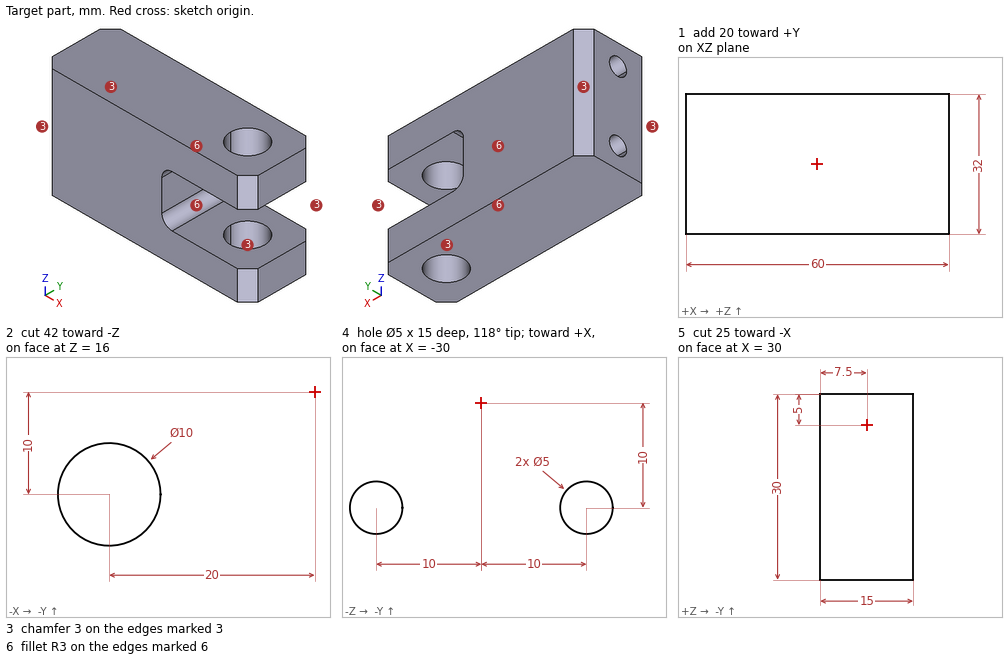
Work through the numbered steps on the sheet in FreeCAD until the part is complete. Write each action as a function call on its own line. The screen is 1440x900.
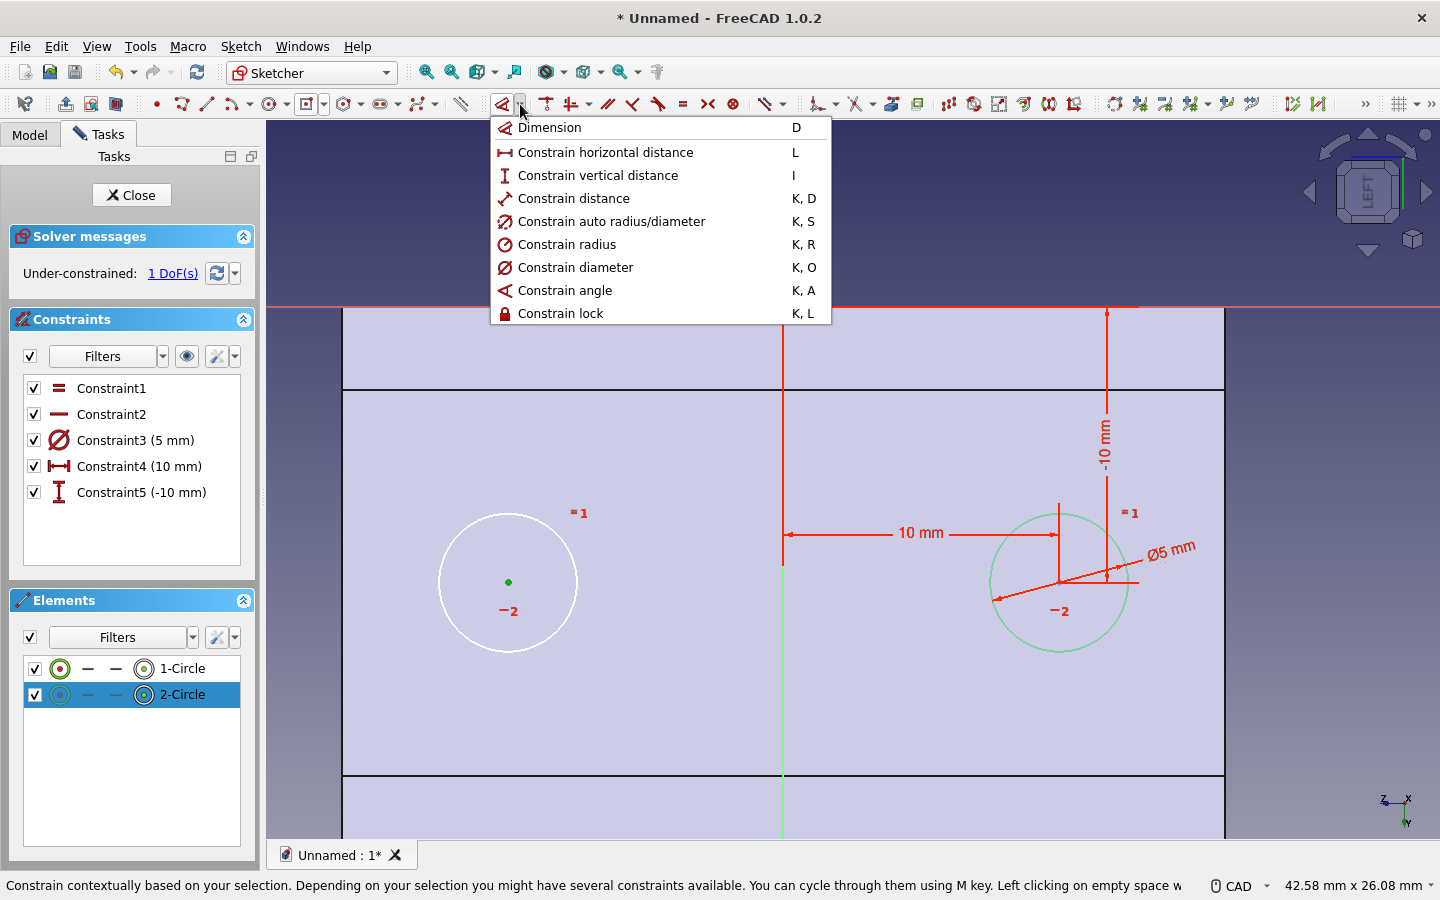
click(661, 152)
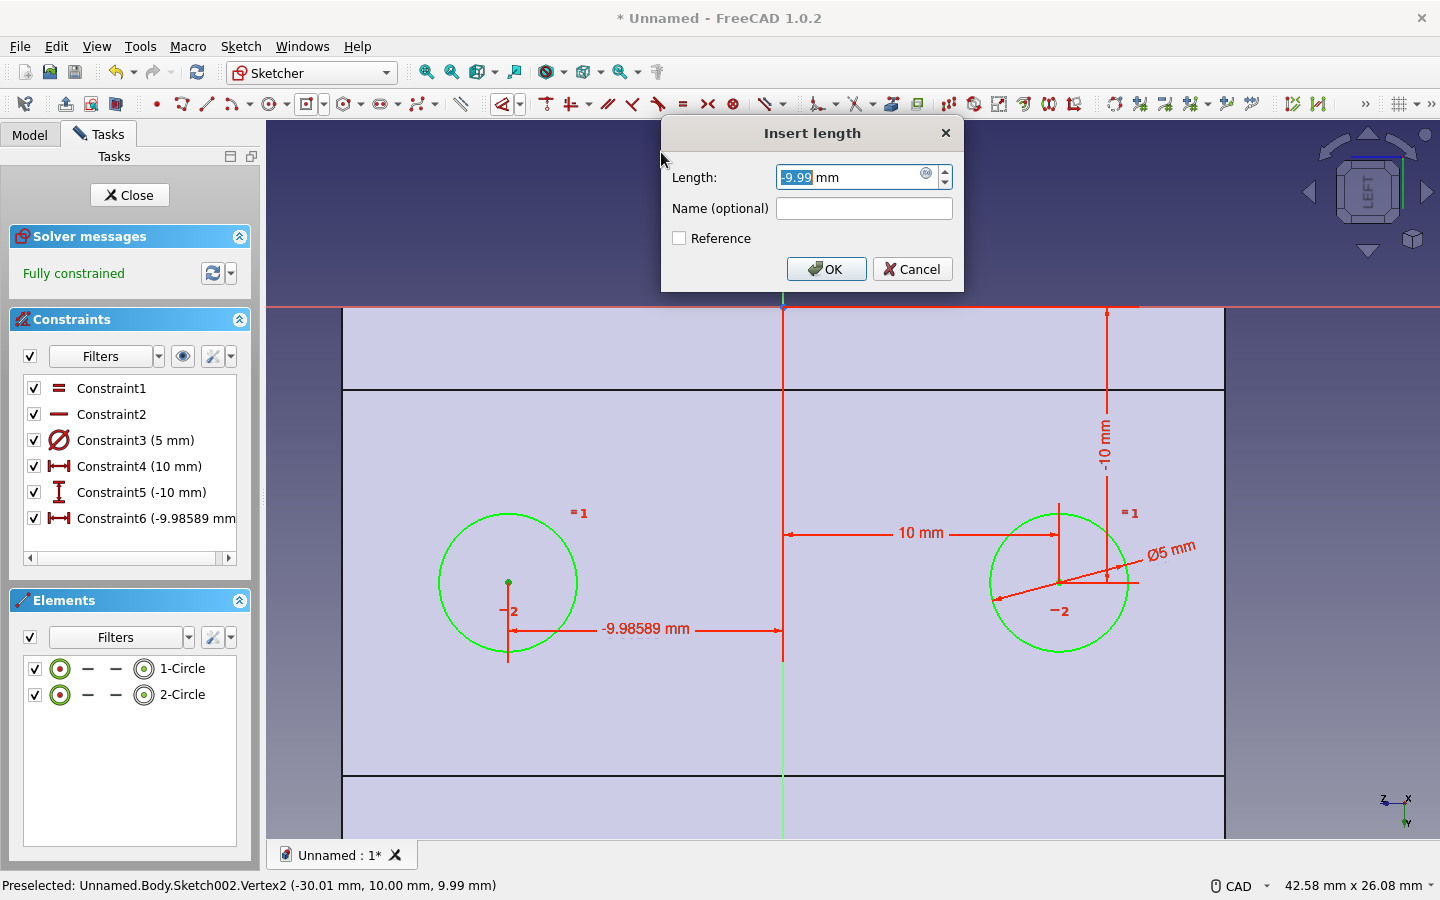
text(-10)
key(Return)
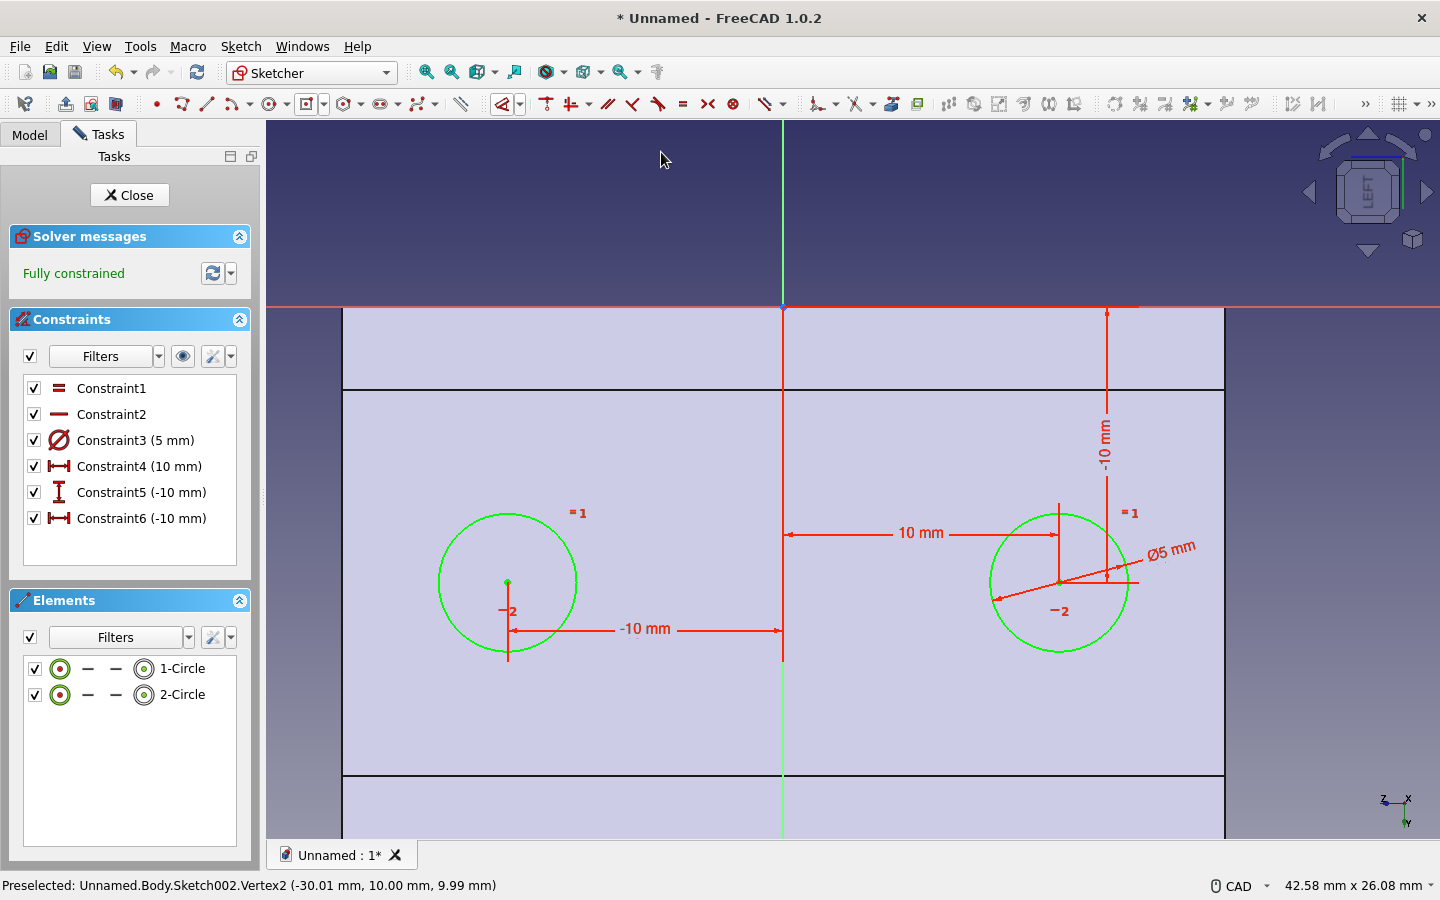
click(130, 195)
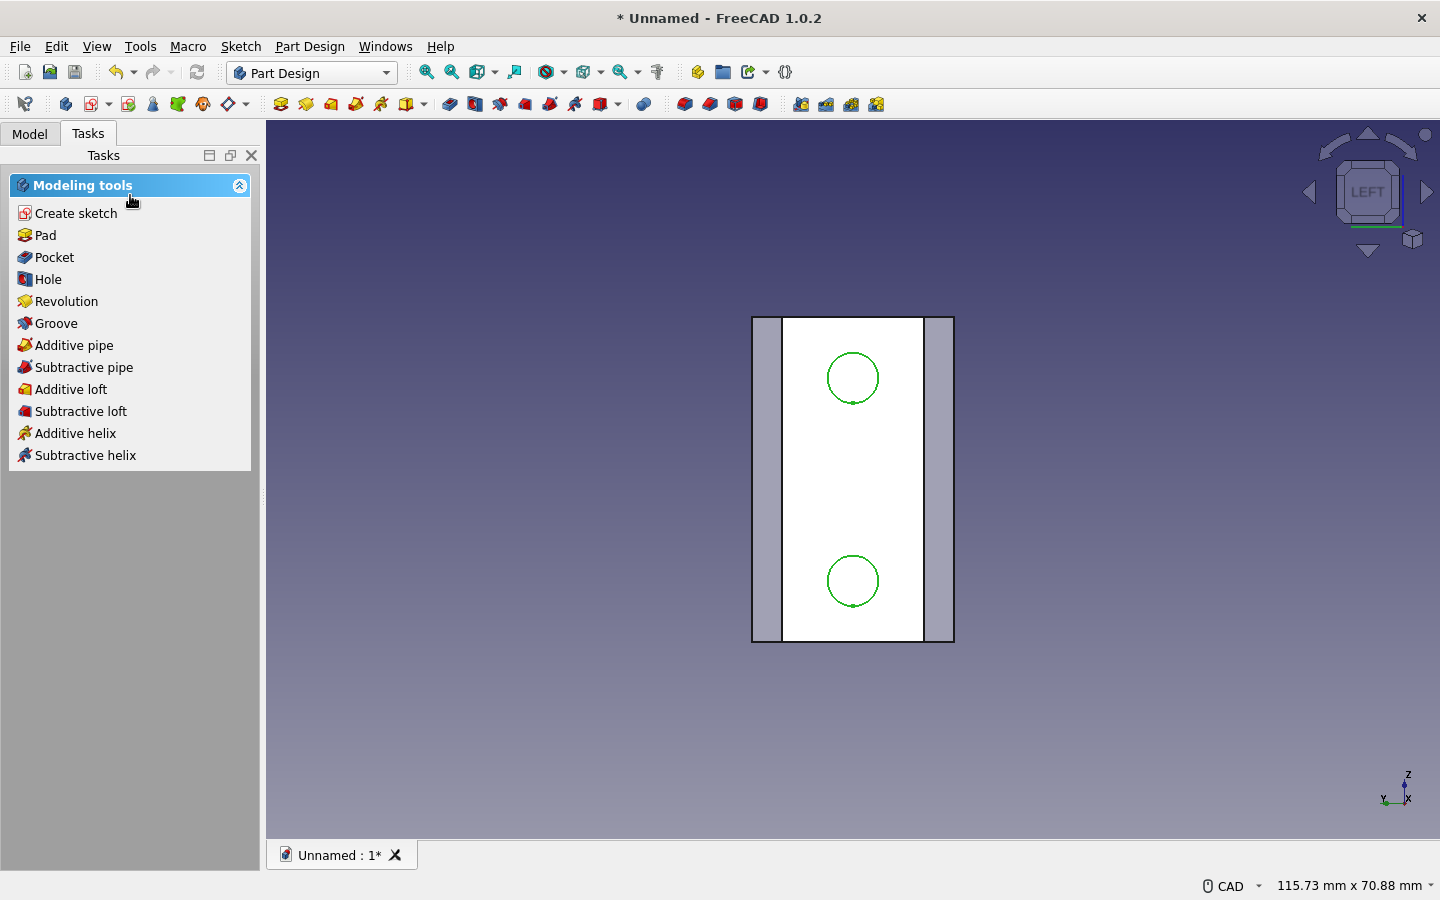
click(475, 104)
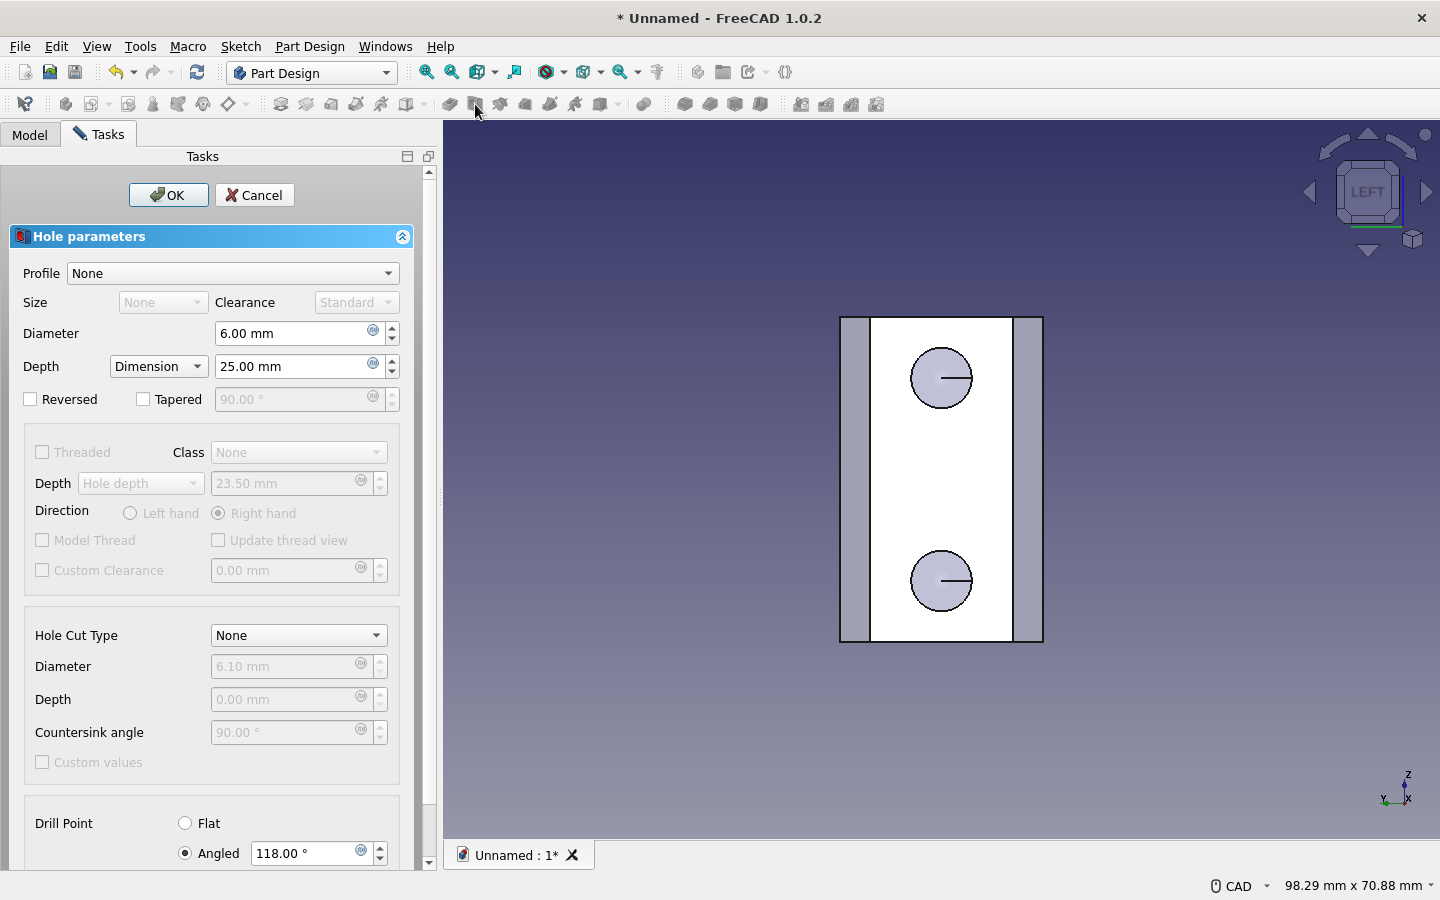
triple_click(300, 334)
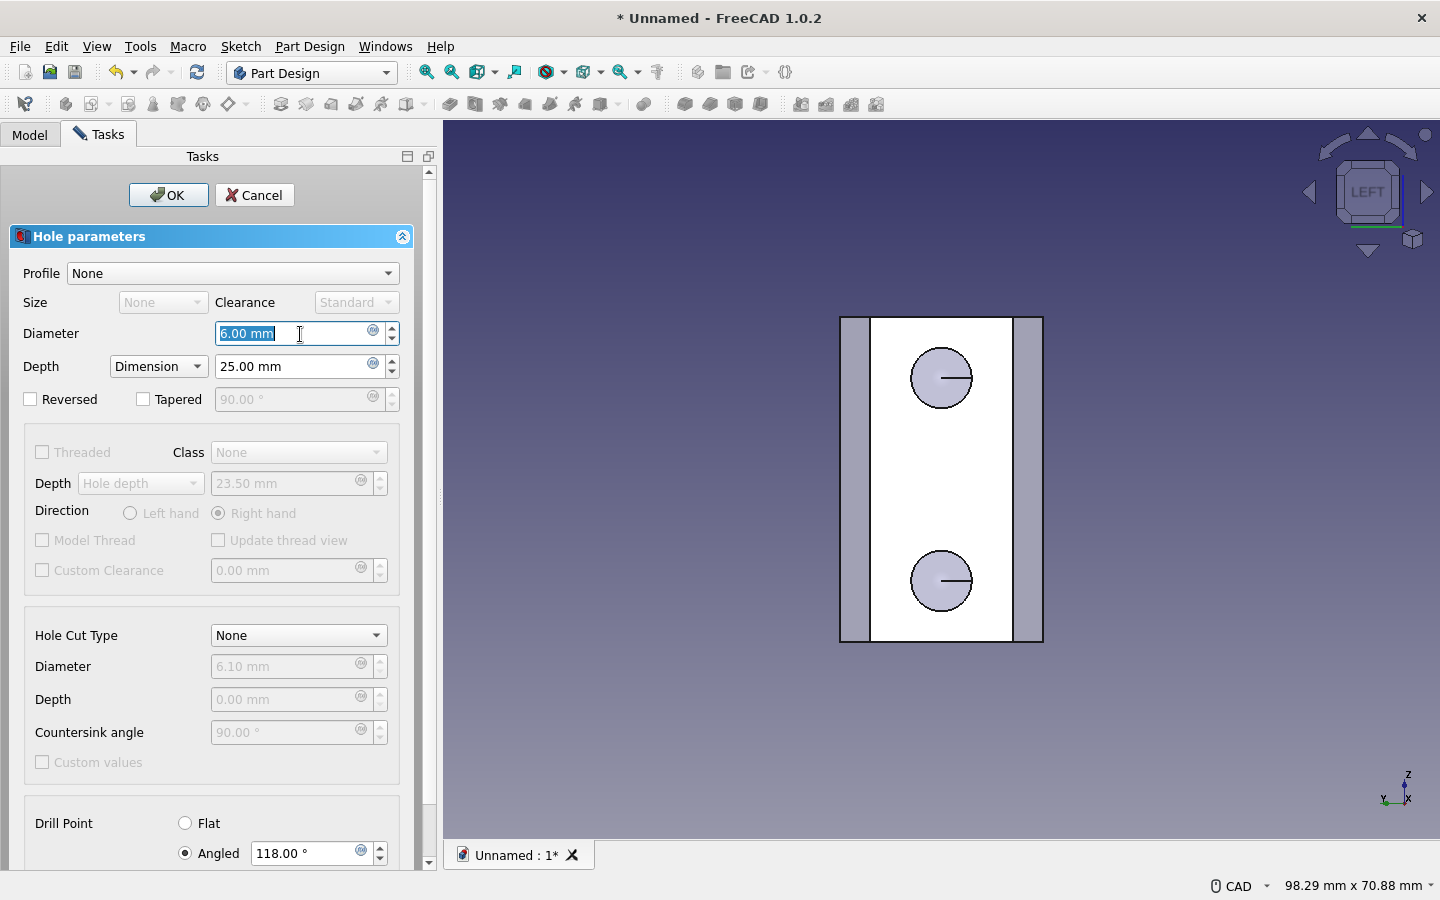
text(5)
key(Tab)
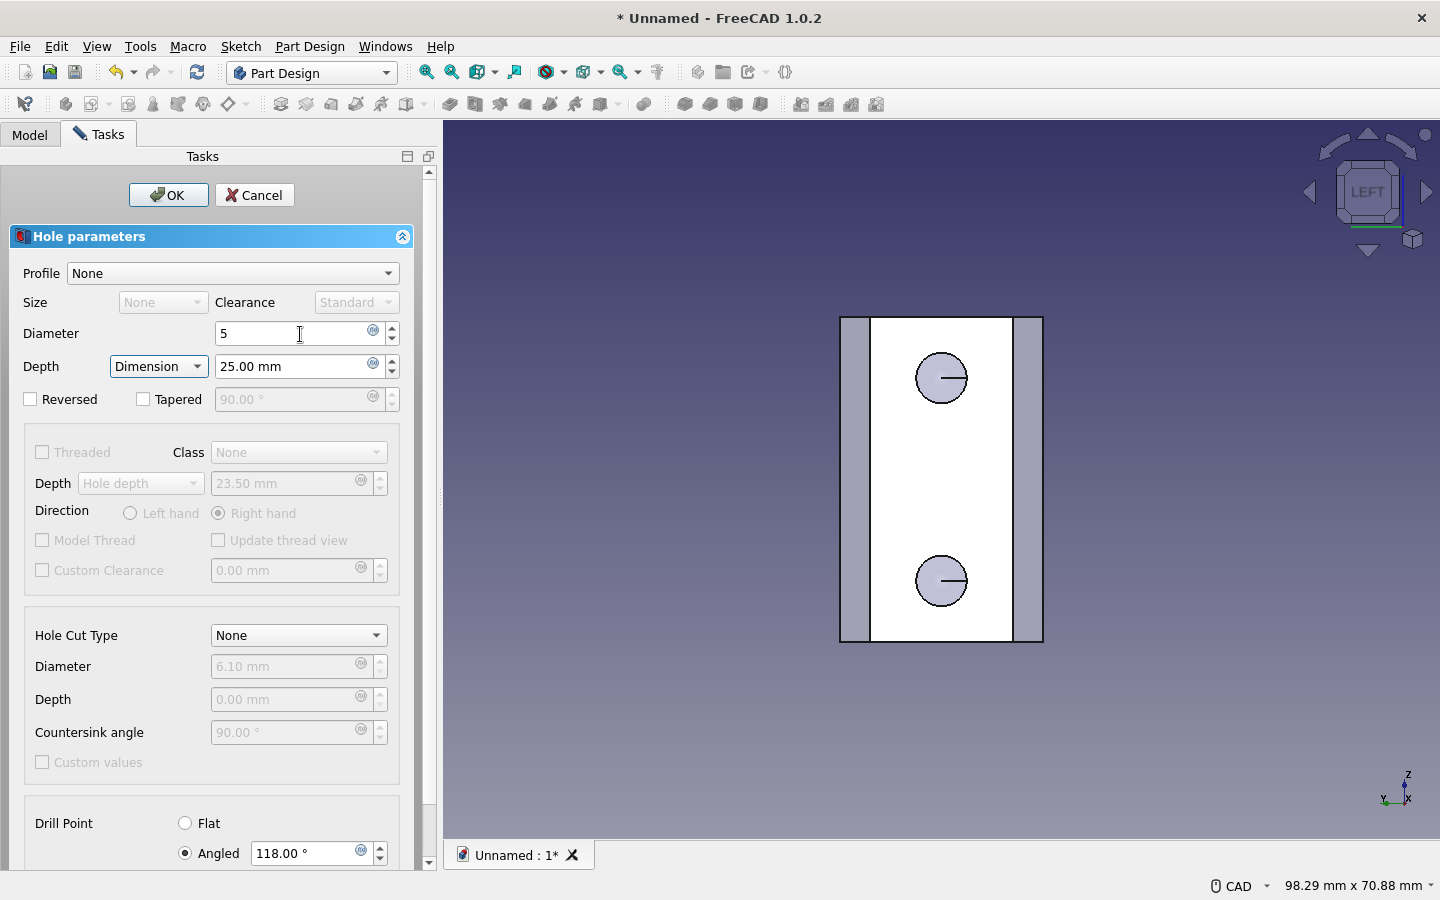
triple_click(300, 366)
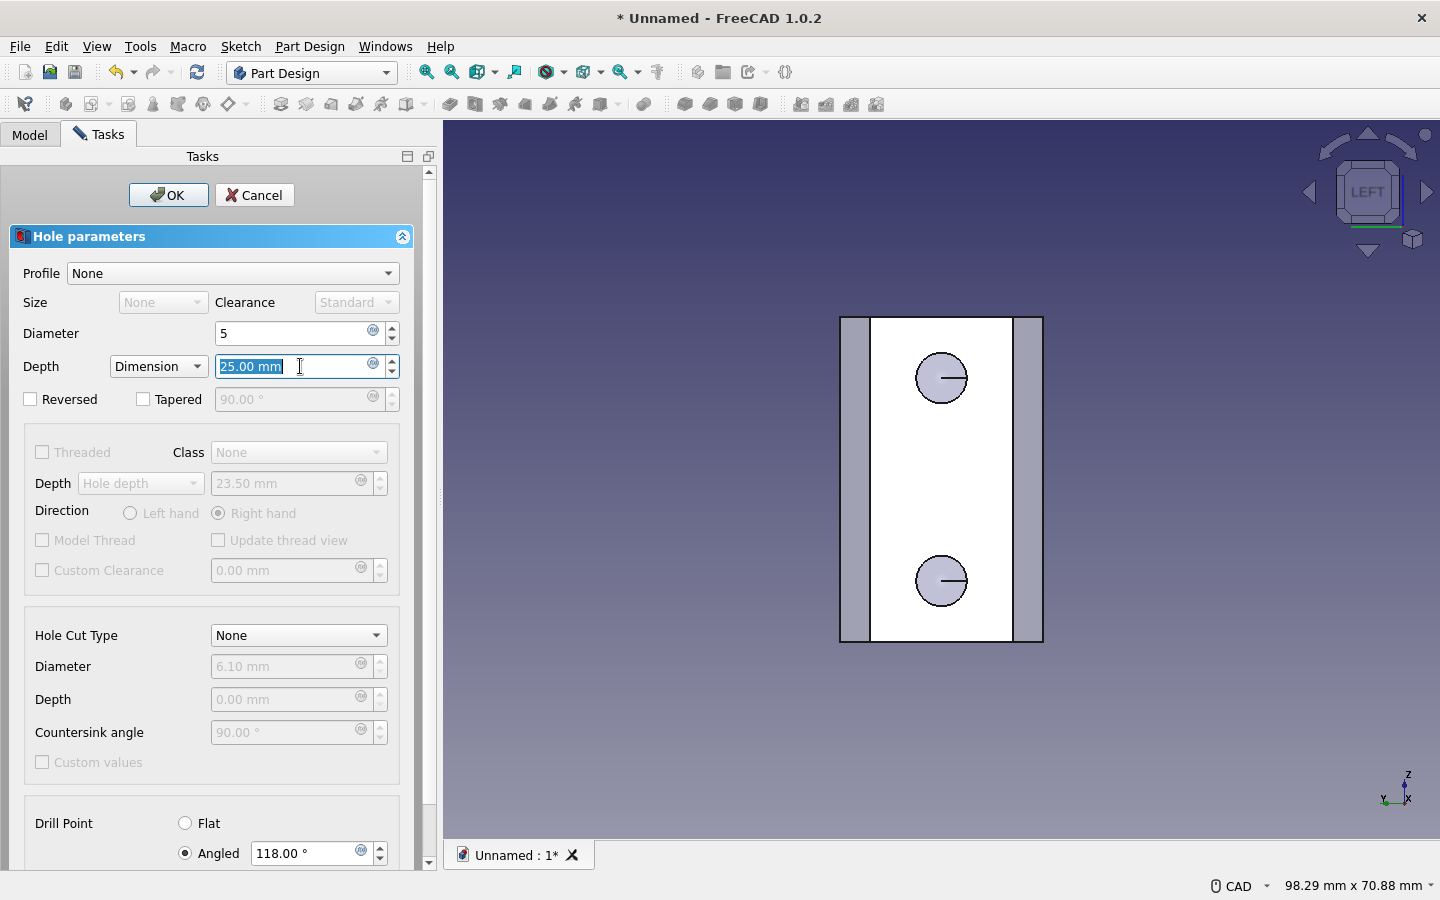
text(15)
key(Tab)